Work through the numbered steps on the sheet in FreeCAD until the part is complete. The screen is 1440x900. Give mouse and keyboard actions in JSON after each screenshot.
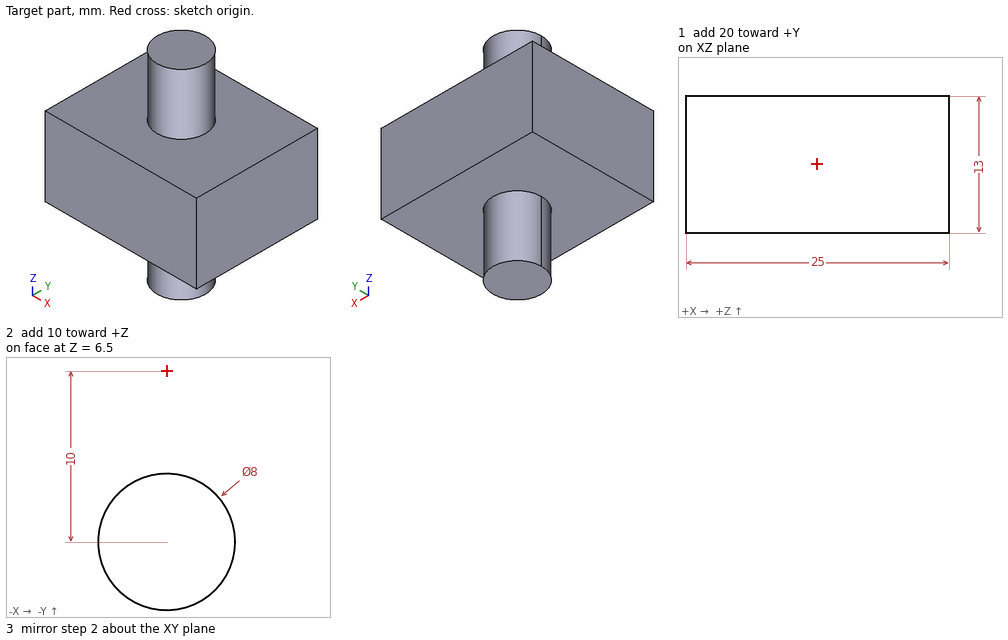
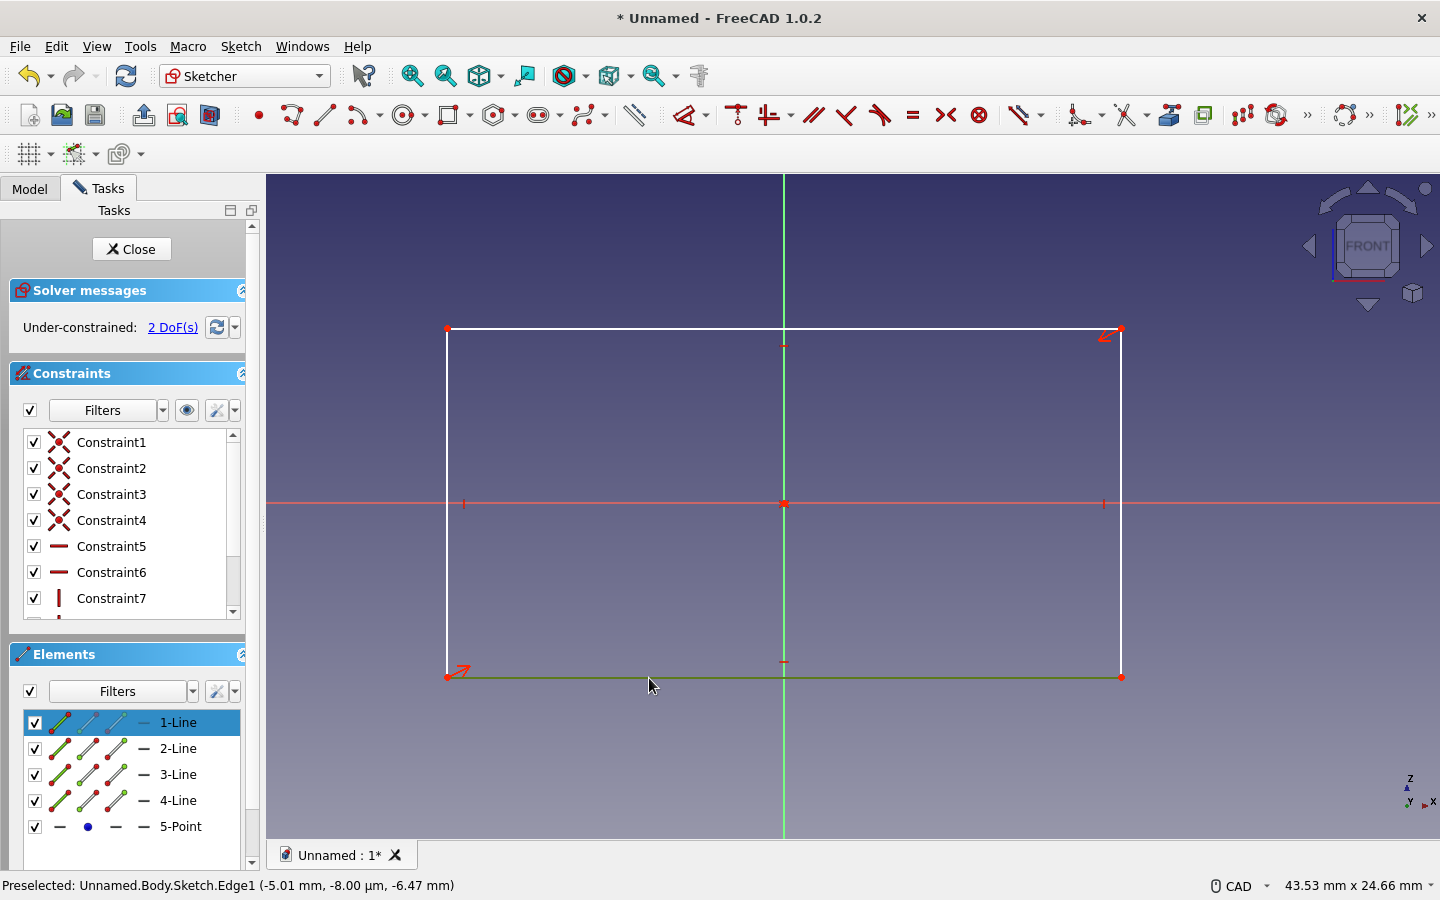
{"action": "key", "text": "l"}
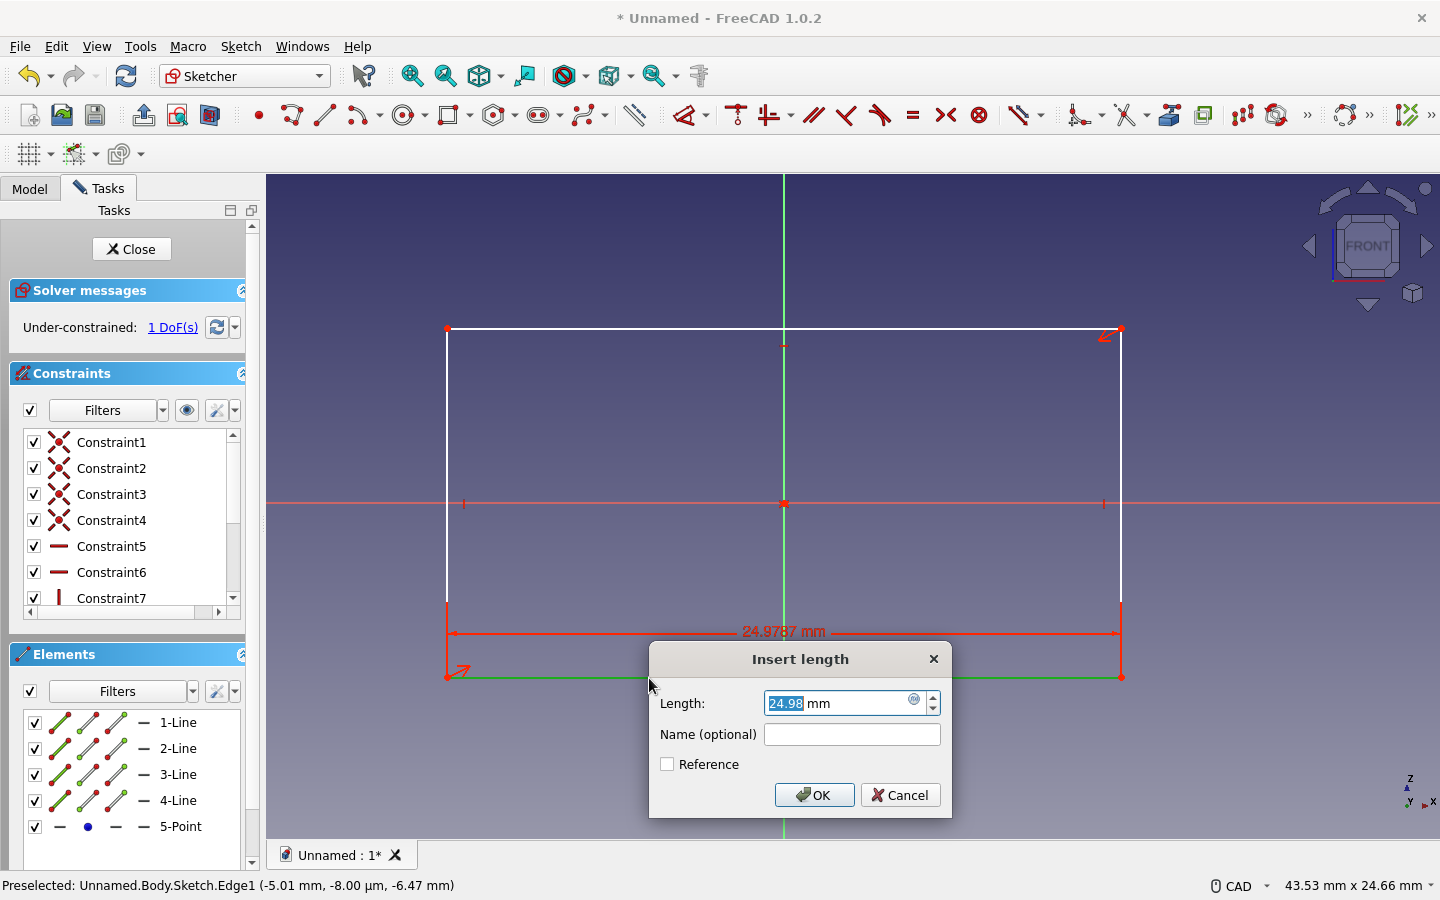
{"action": "type", "text": "25"}
{"action": "key", "text": "Return"}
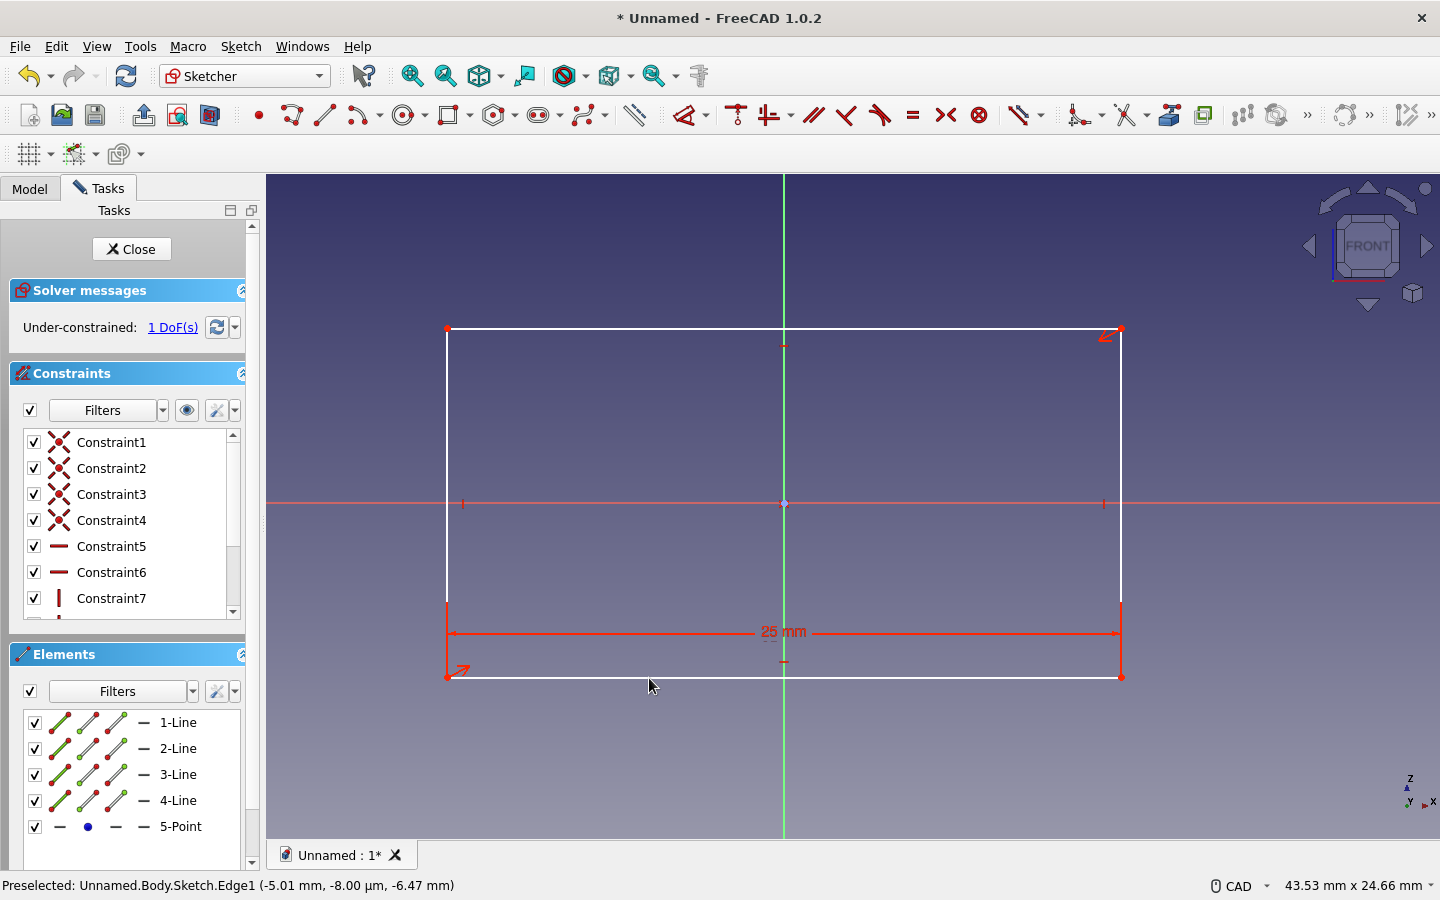
{"action": "left_click", "coordinate": [1121, 573]}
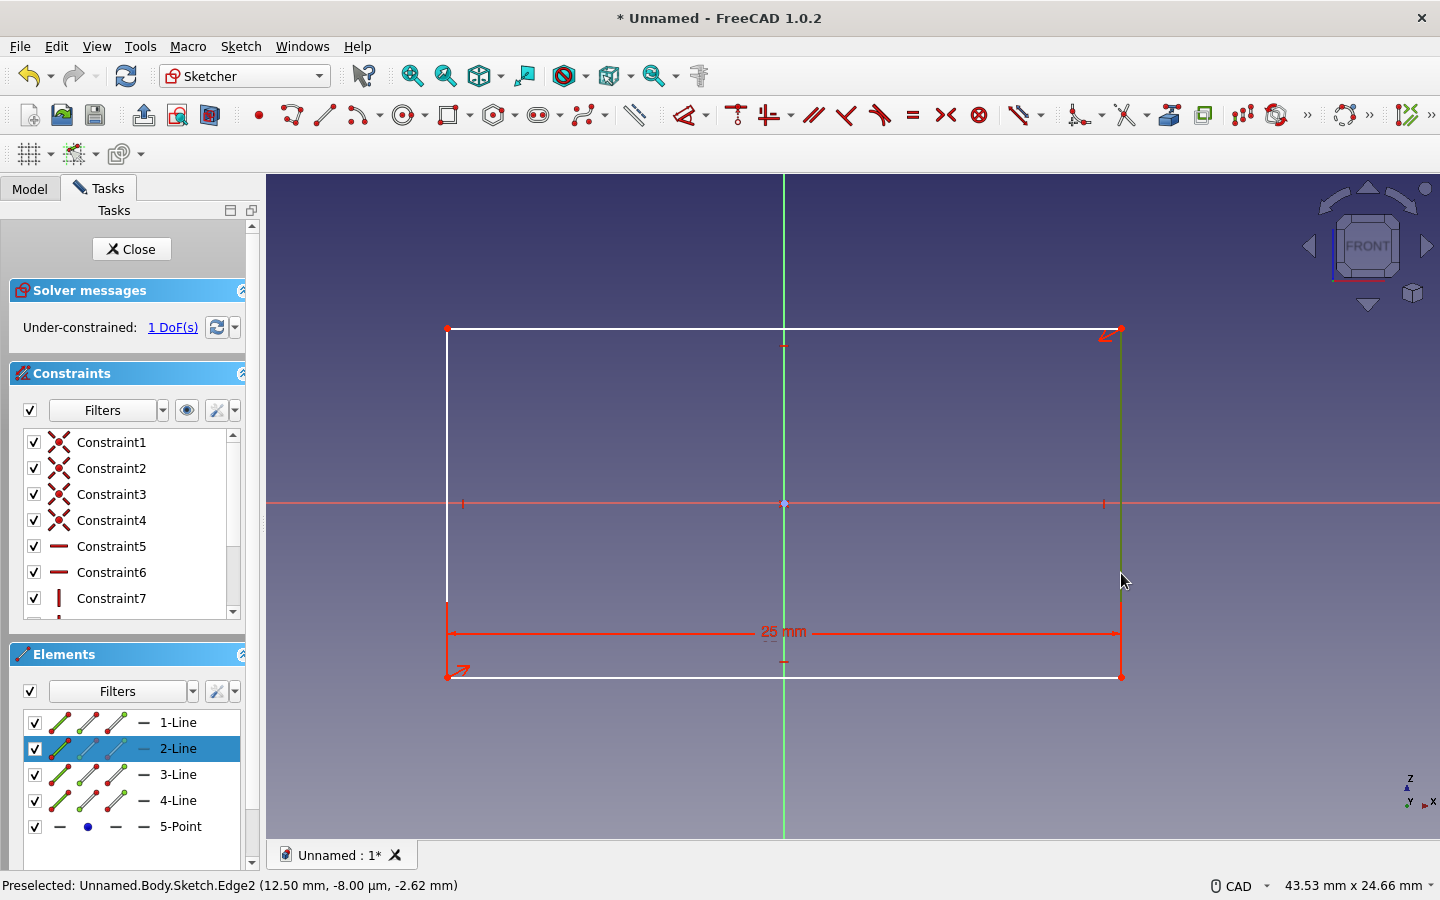
{"action": "left_click", "coordinate": [706, 116]}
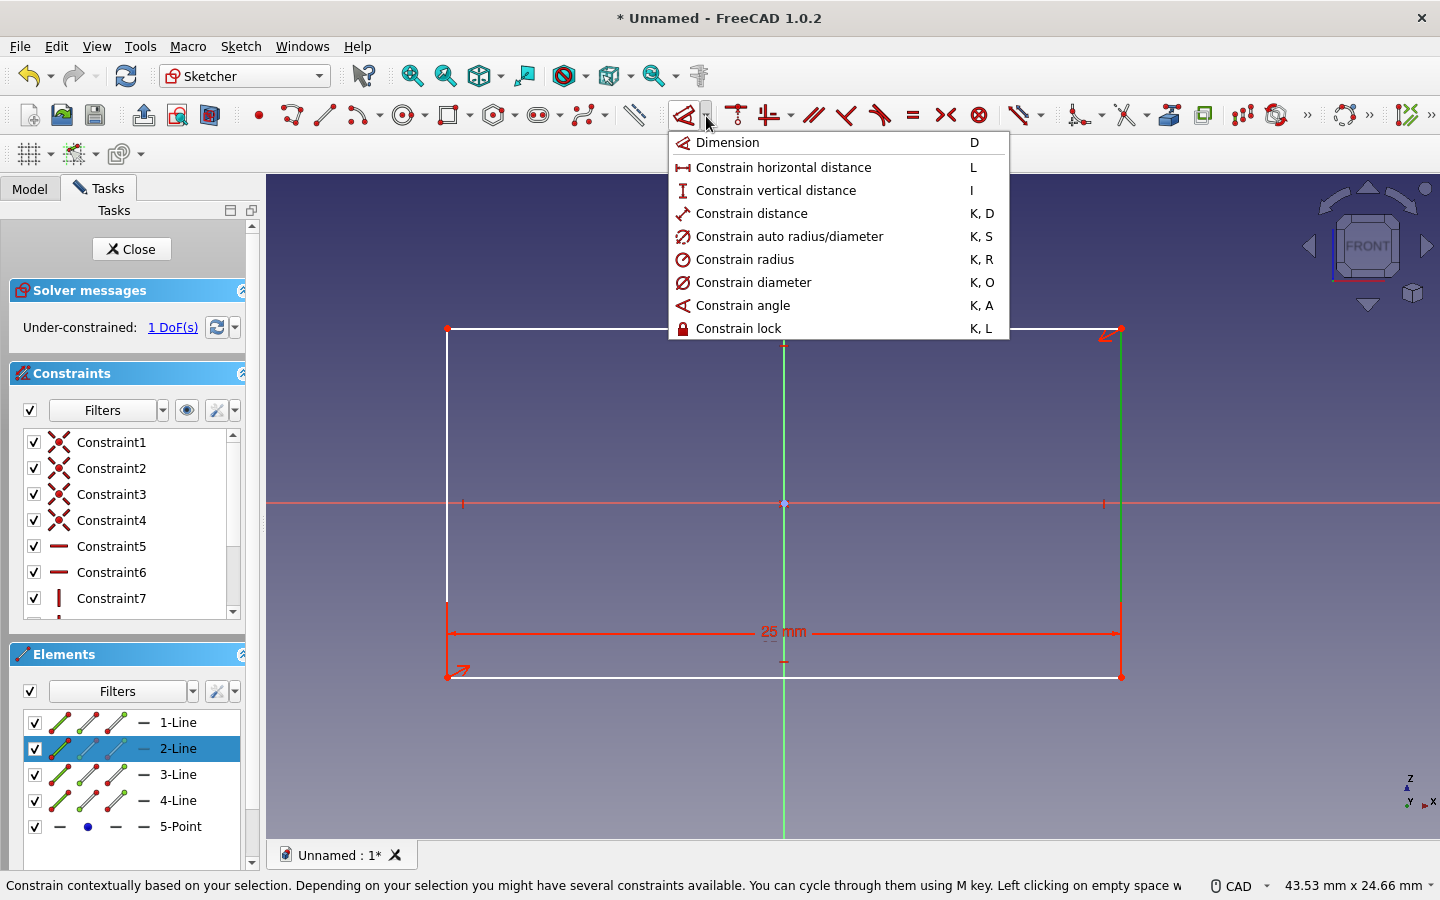
{"action": "left_click", "coordinate": [839, 190]}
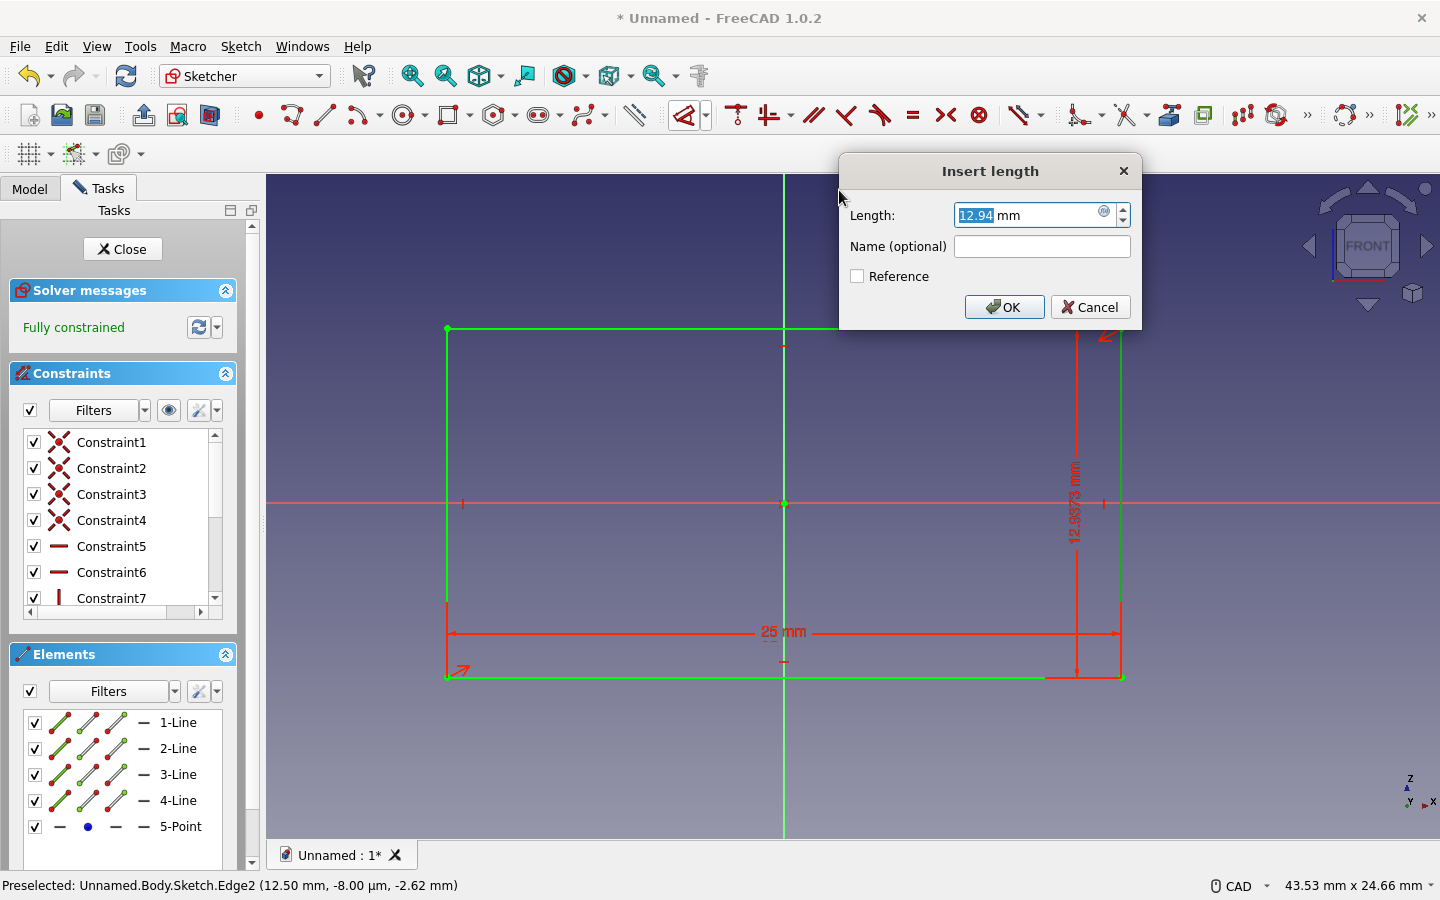
{"action": "type", "text": "13"}
{"action": "key", "text": "Return"}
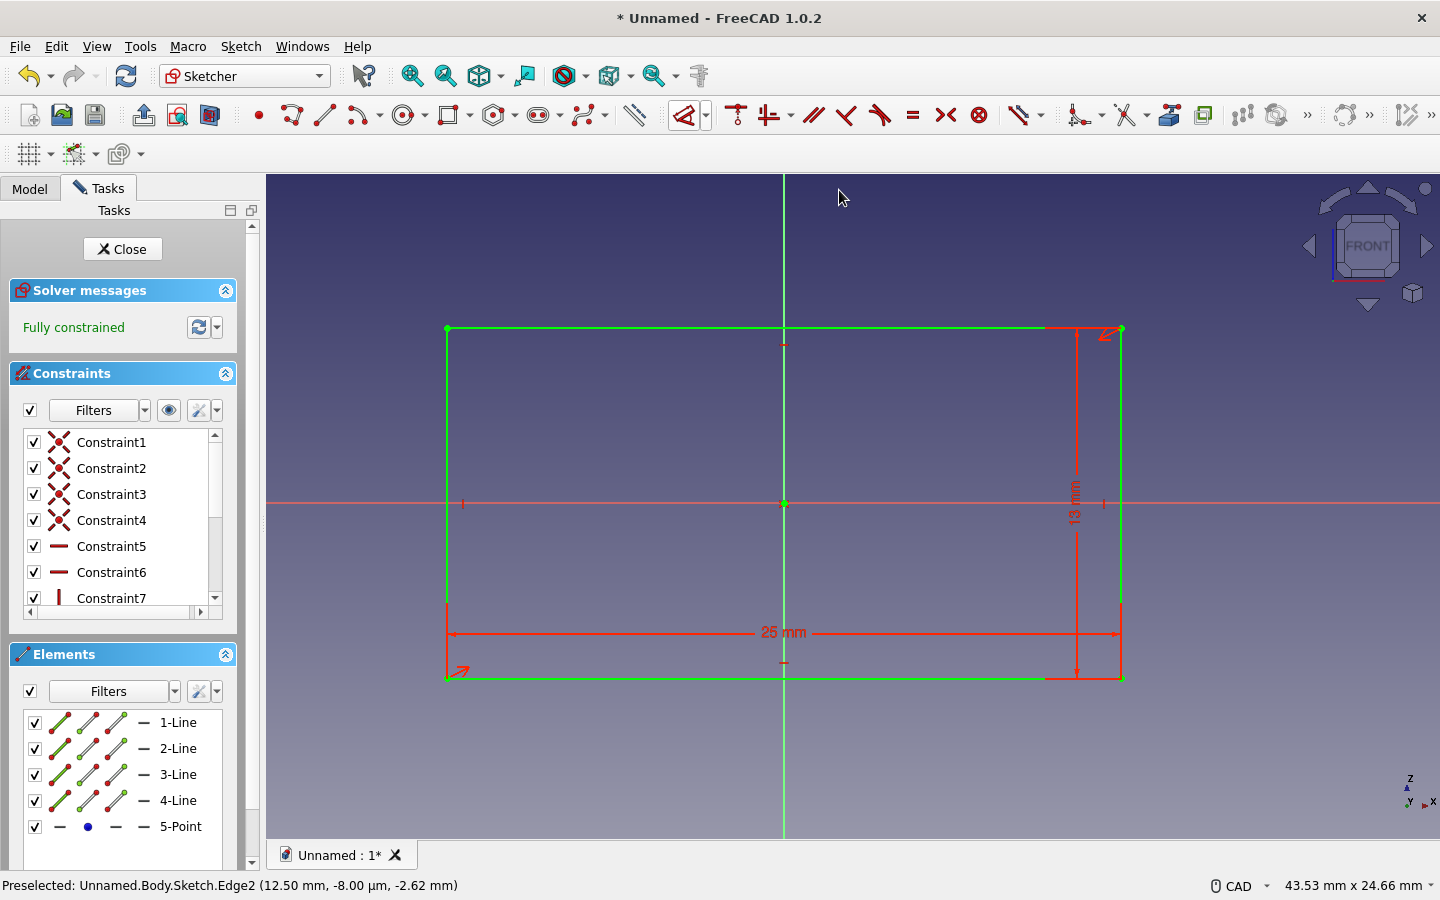
{"action": "left_click", "coordinate": [123, 249]}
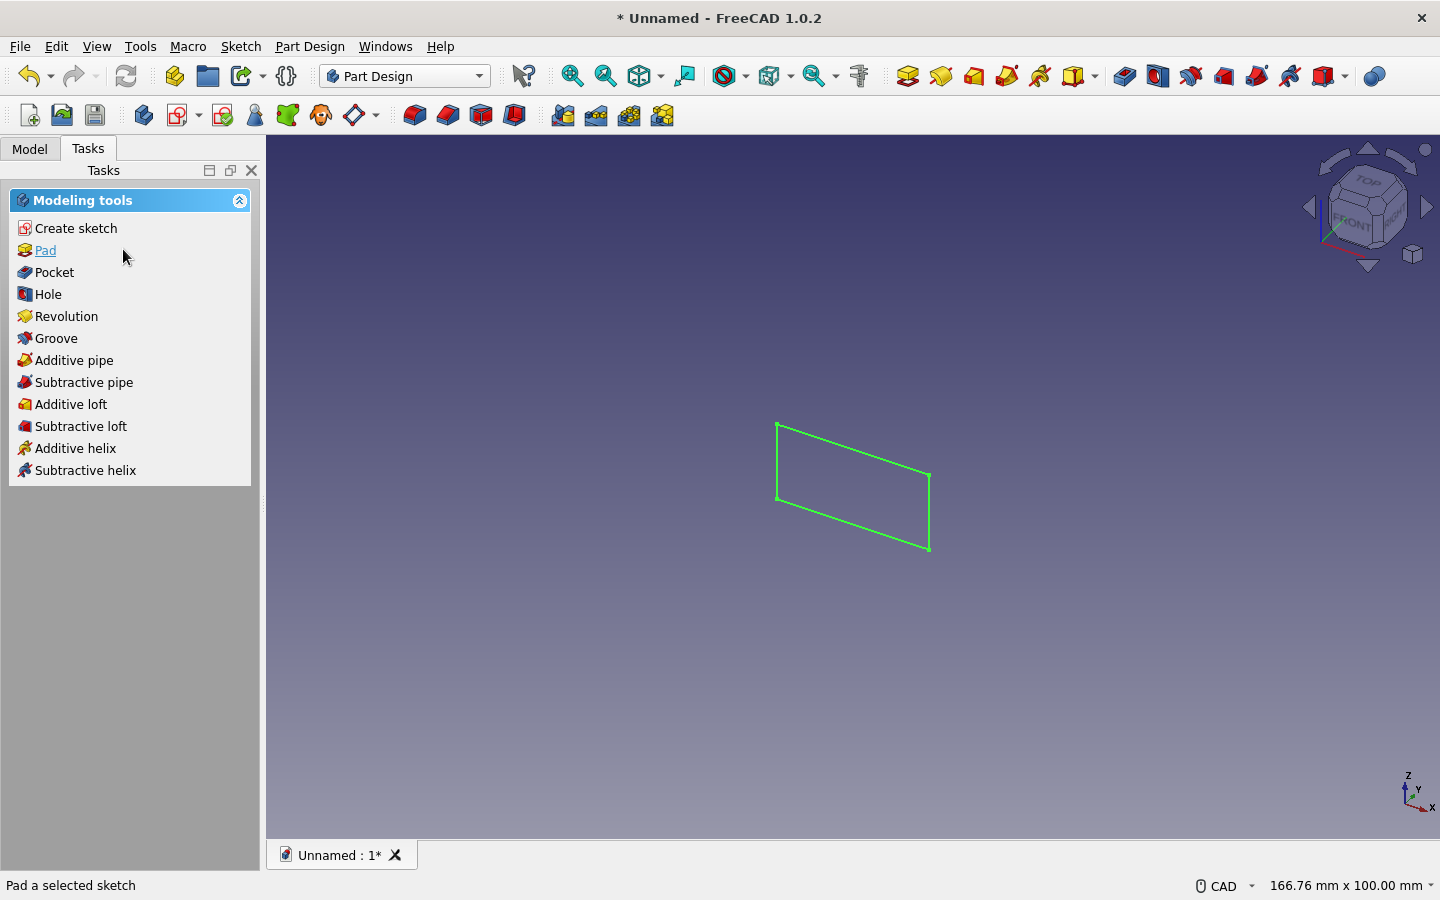
{"action": "left_click", "coordinate": [908, 76]}